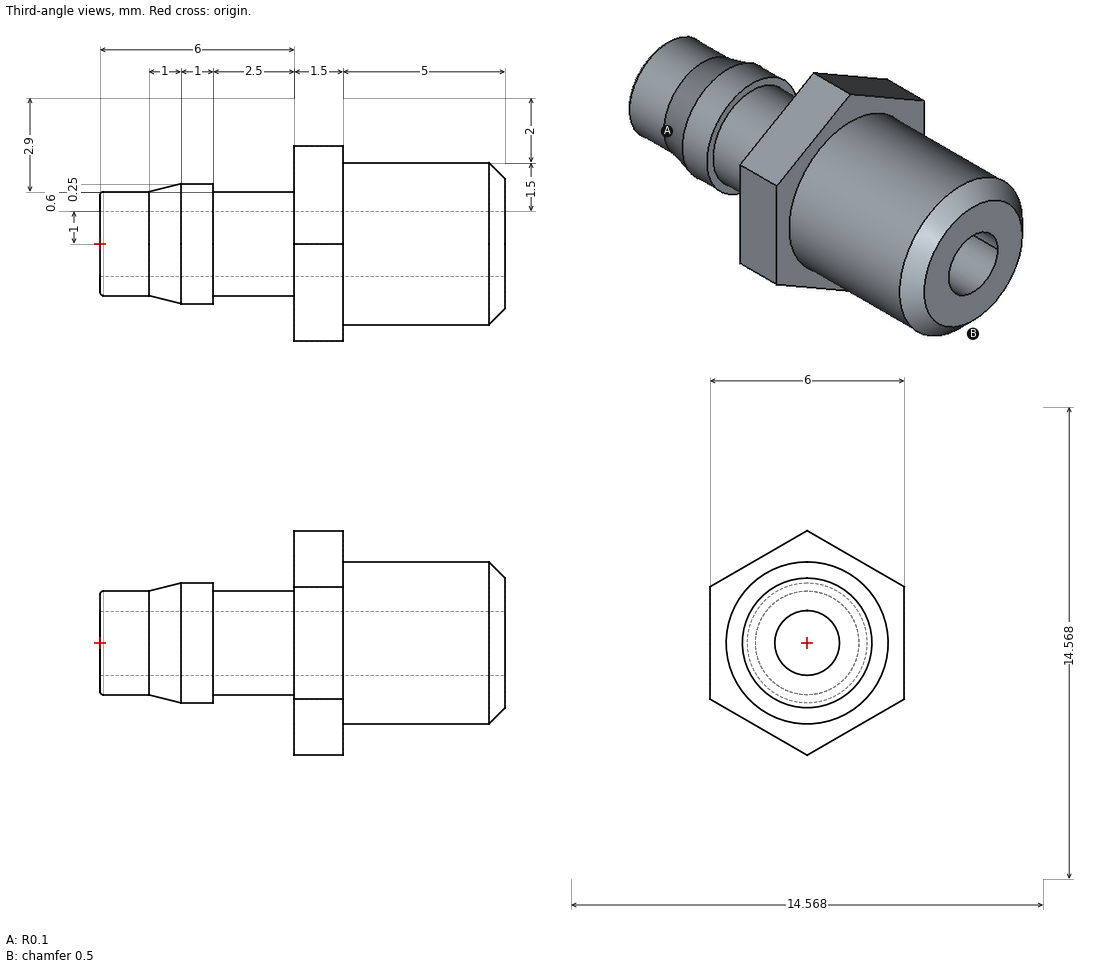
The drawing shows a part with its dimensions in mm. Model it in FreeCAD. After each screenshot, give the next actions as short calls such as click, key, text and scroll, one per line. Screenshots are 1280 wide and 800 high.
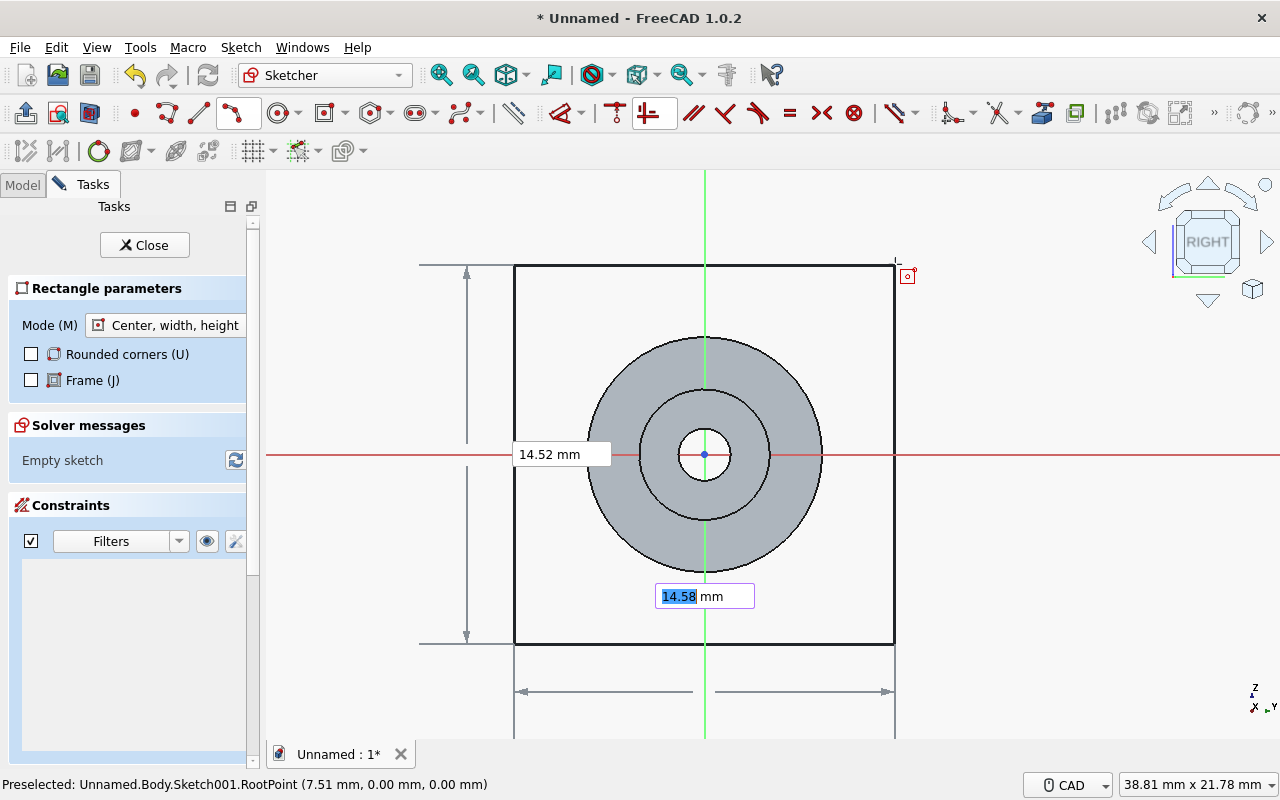
text(14.568)
key(Tab)
text(14.568)
key(Return)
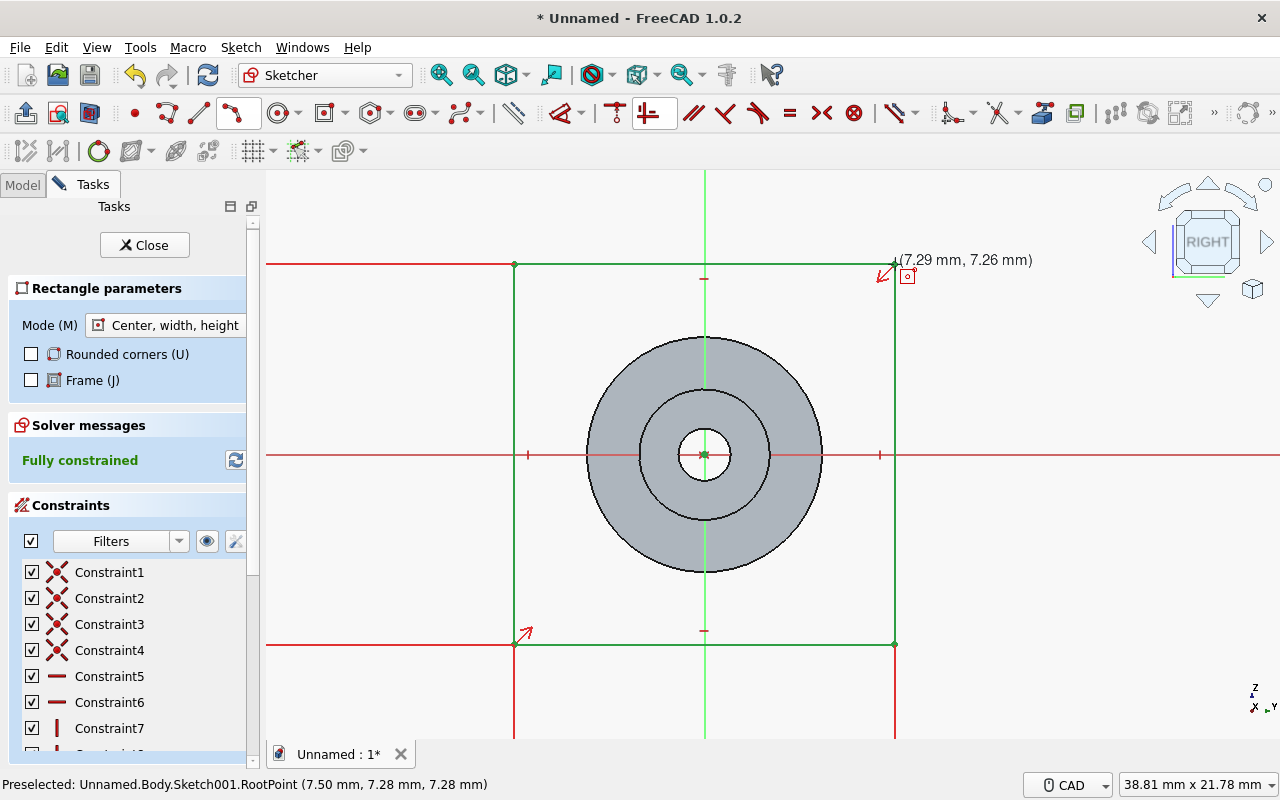
click(370, 114)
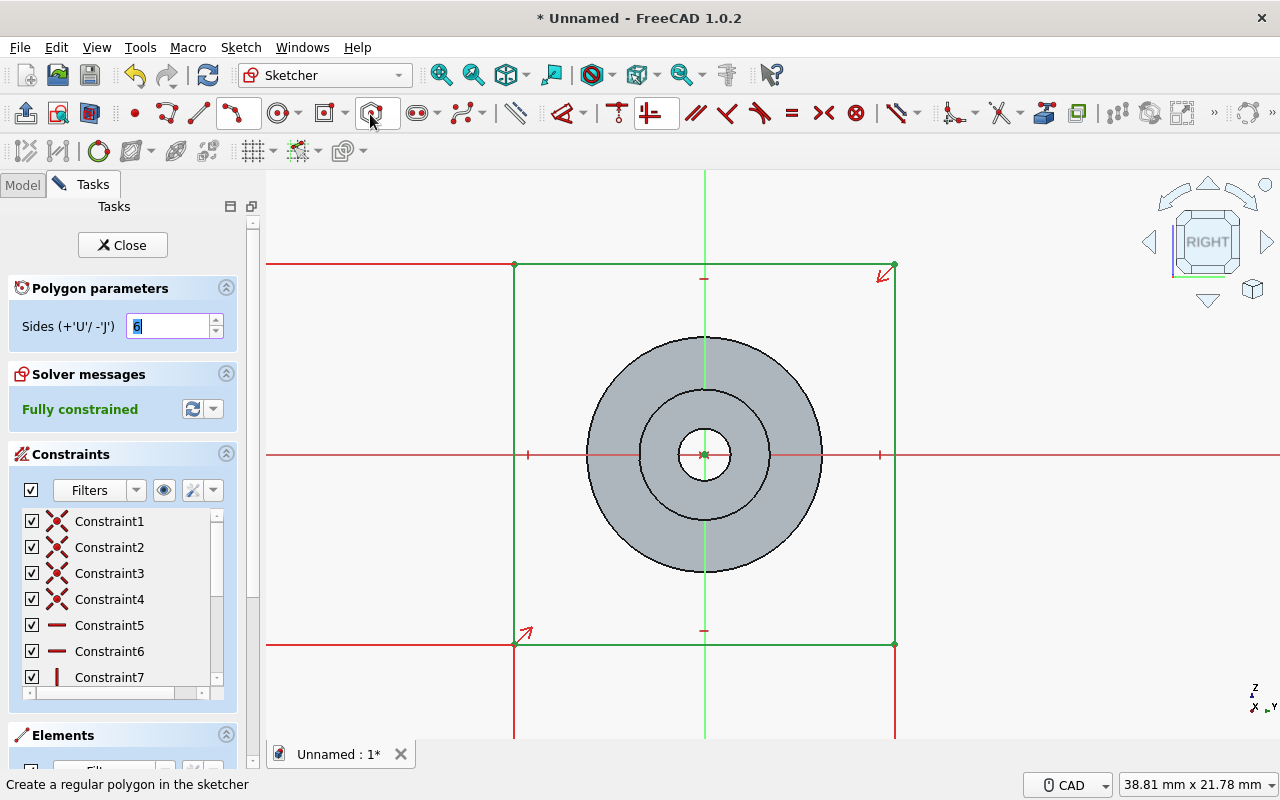
click(705, 455)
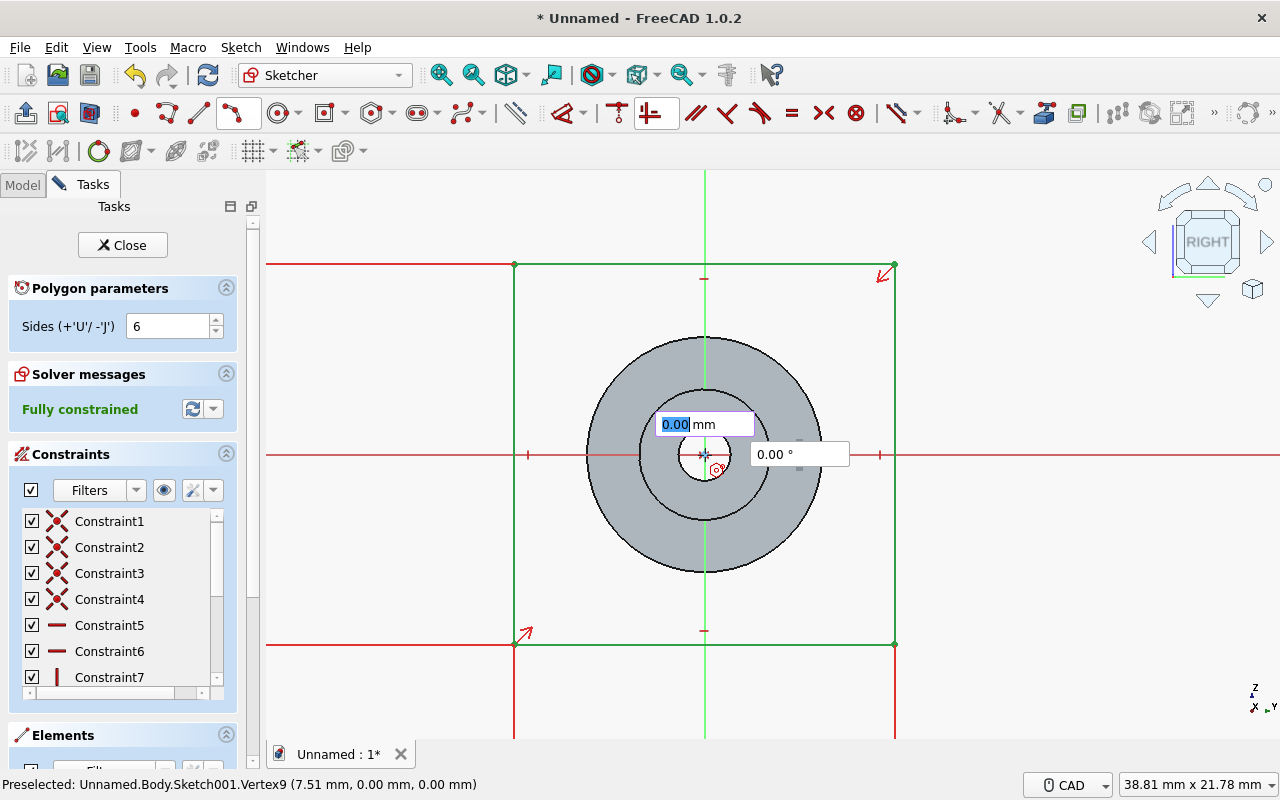
click(705, 545)
right_click(705, 545)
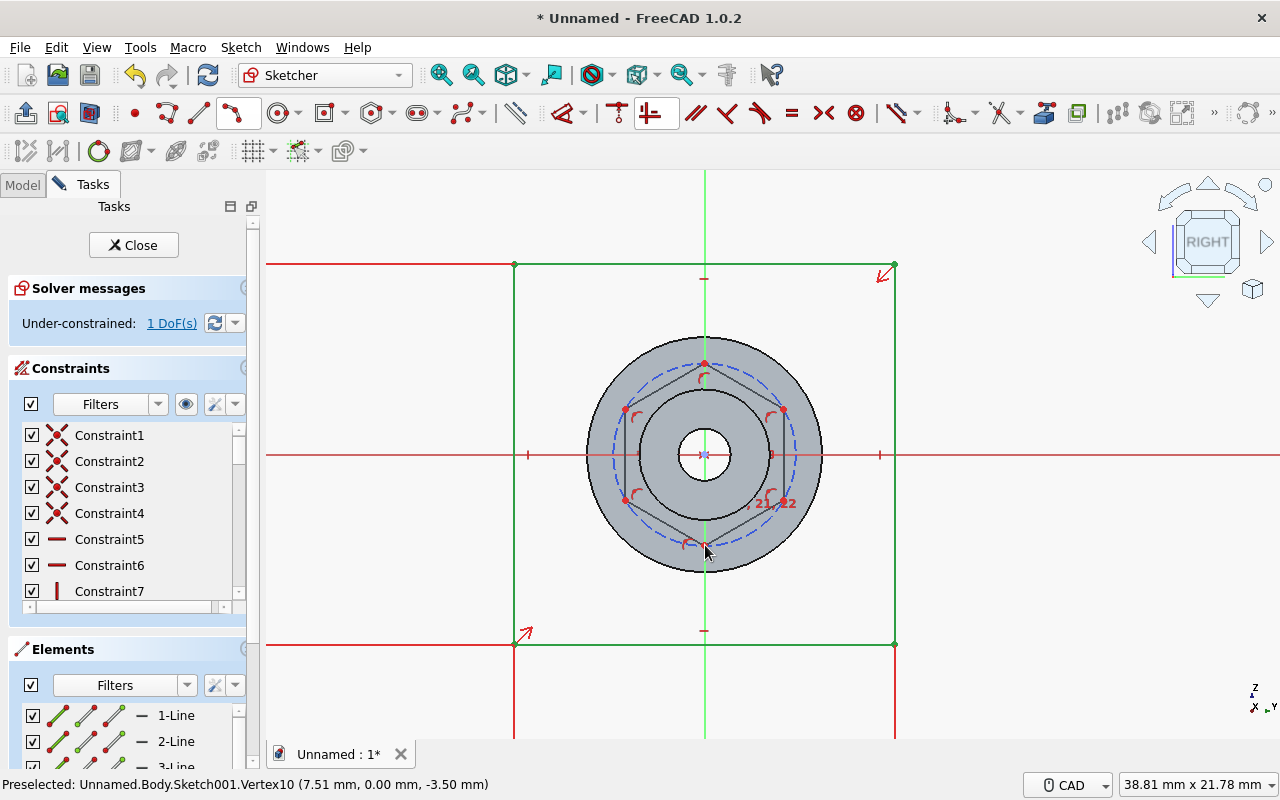
key(d)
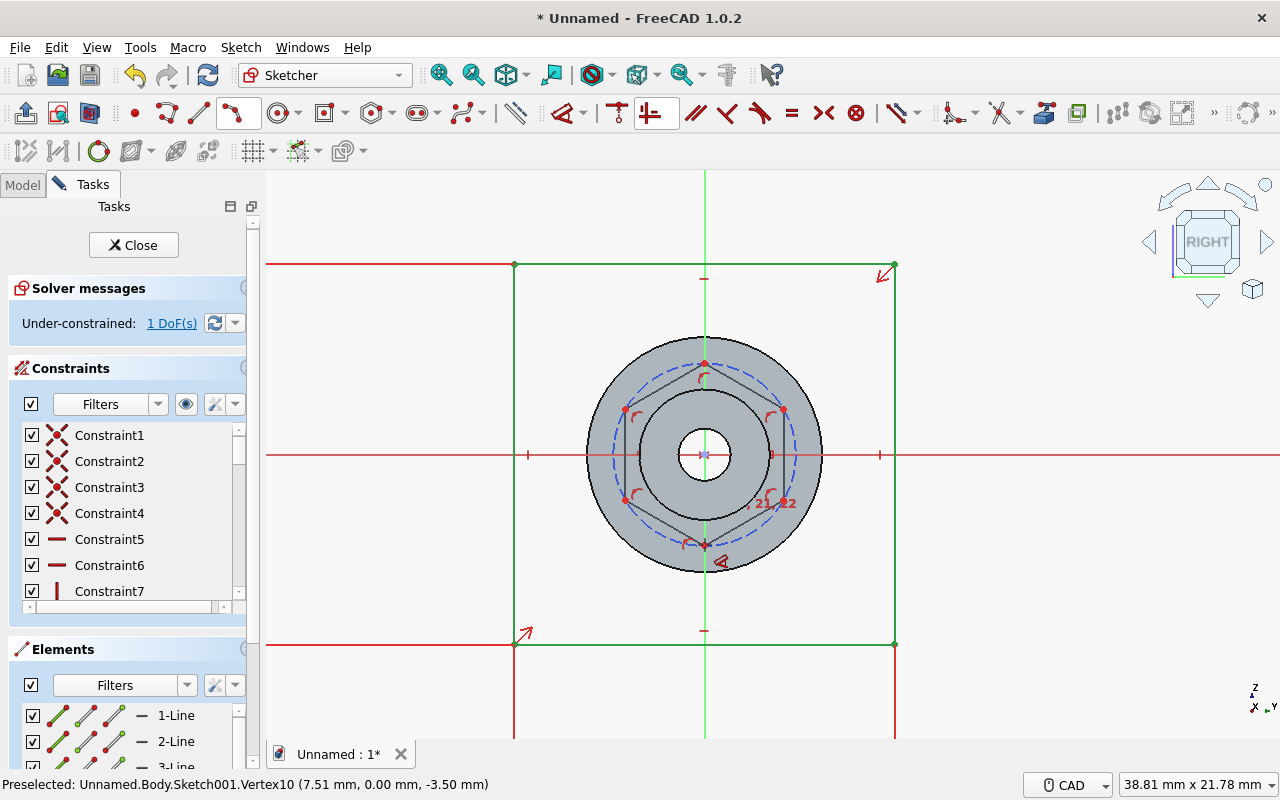
click(625, 409)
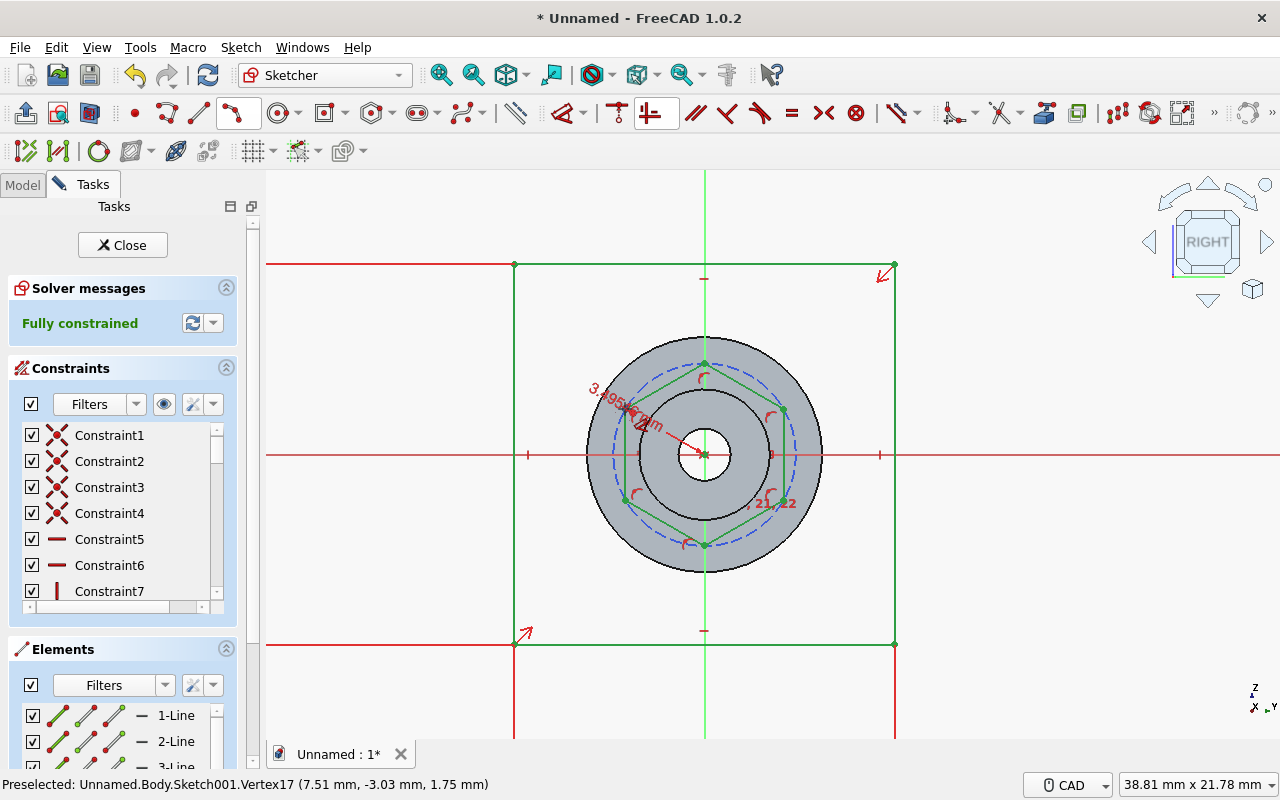
click(784, 500)
click(668, 558)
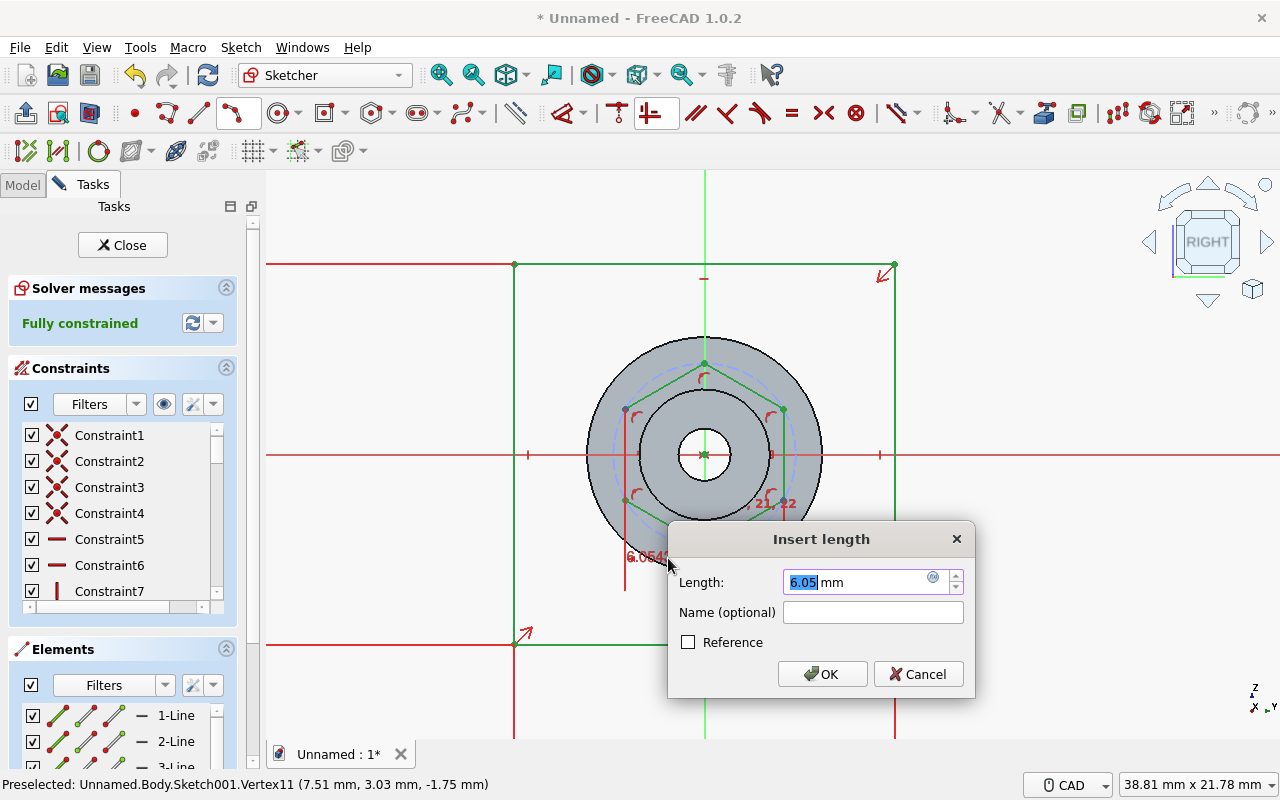
text(6)
key(Return)
key(Escape)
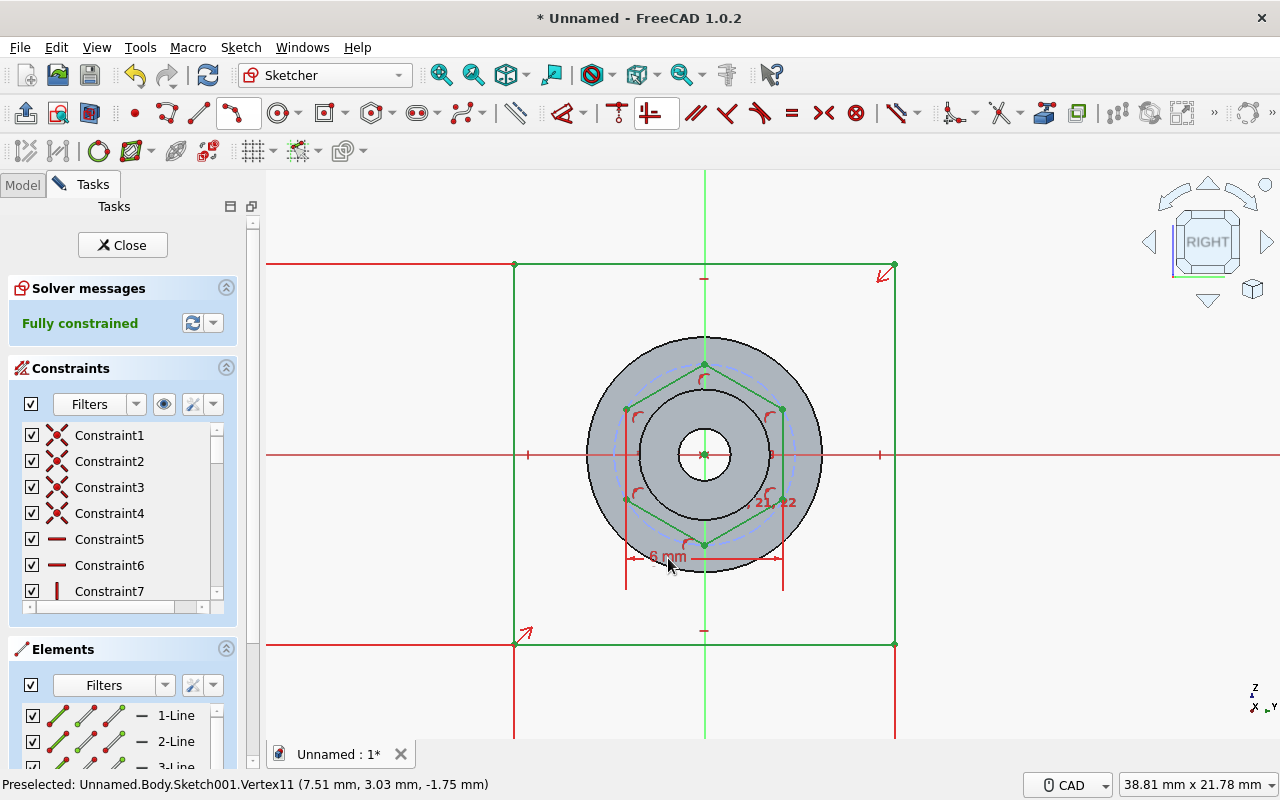
click(123, 245)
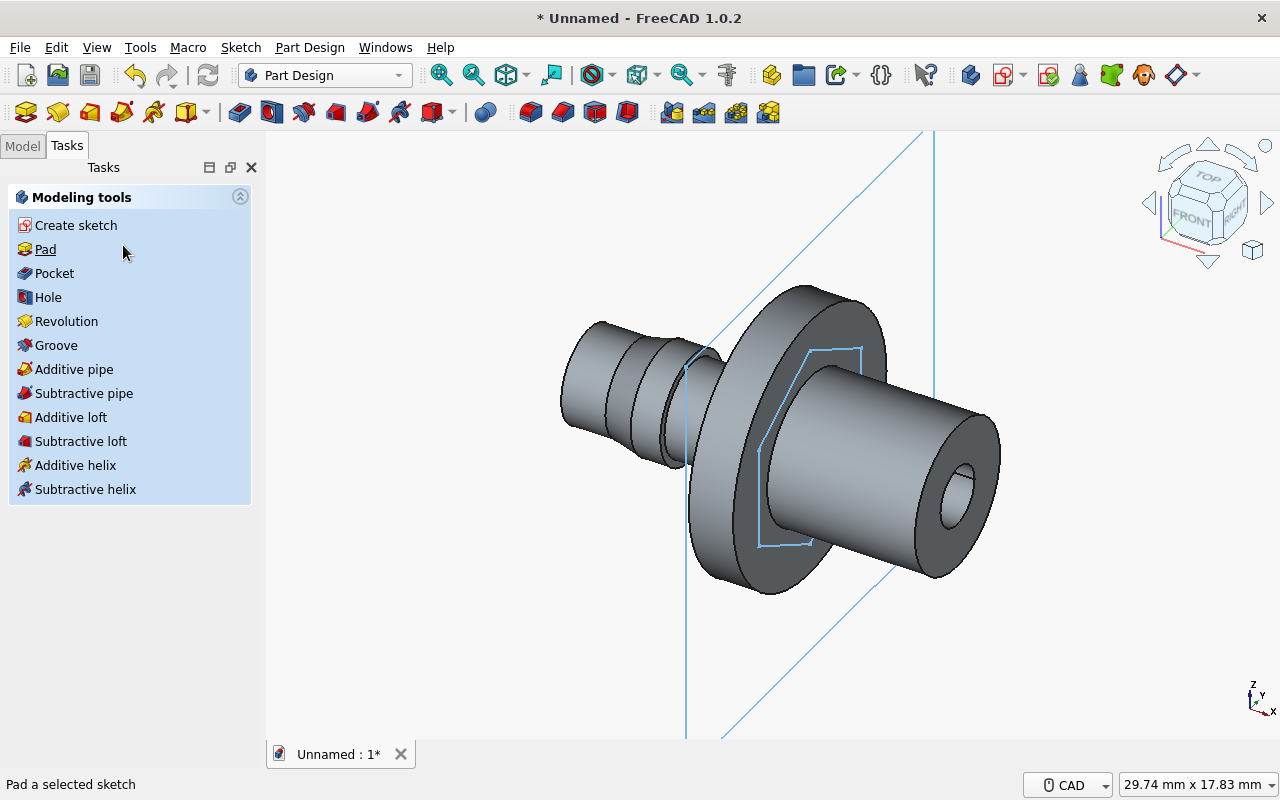
click(240, 112)